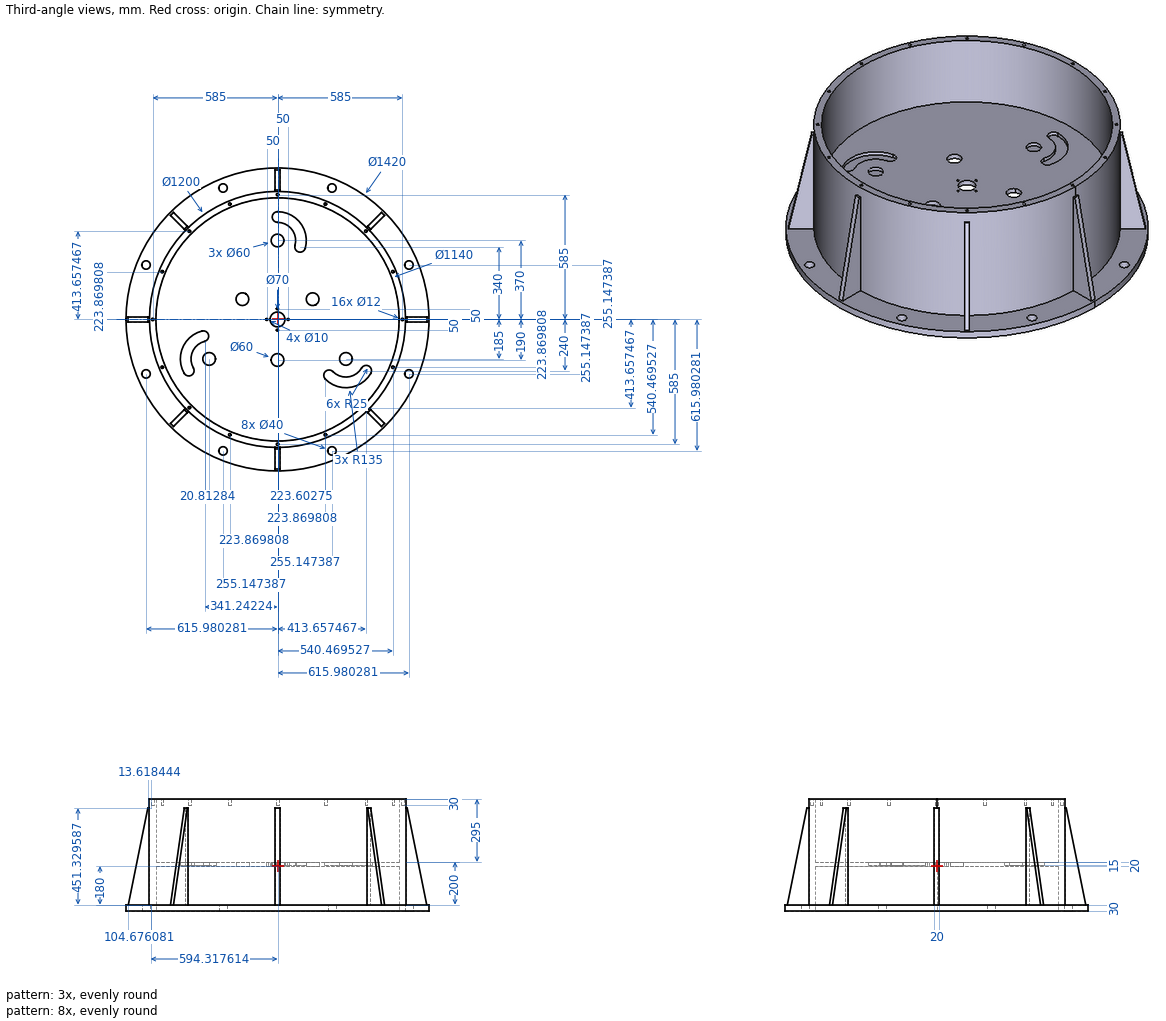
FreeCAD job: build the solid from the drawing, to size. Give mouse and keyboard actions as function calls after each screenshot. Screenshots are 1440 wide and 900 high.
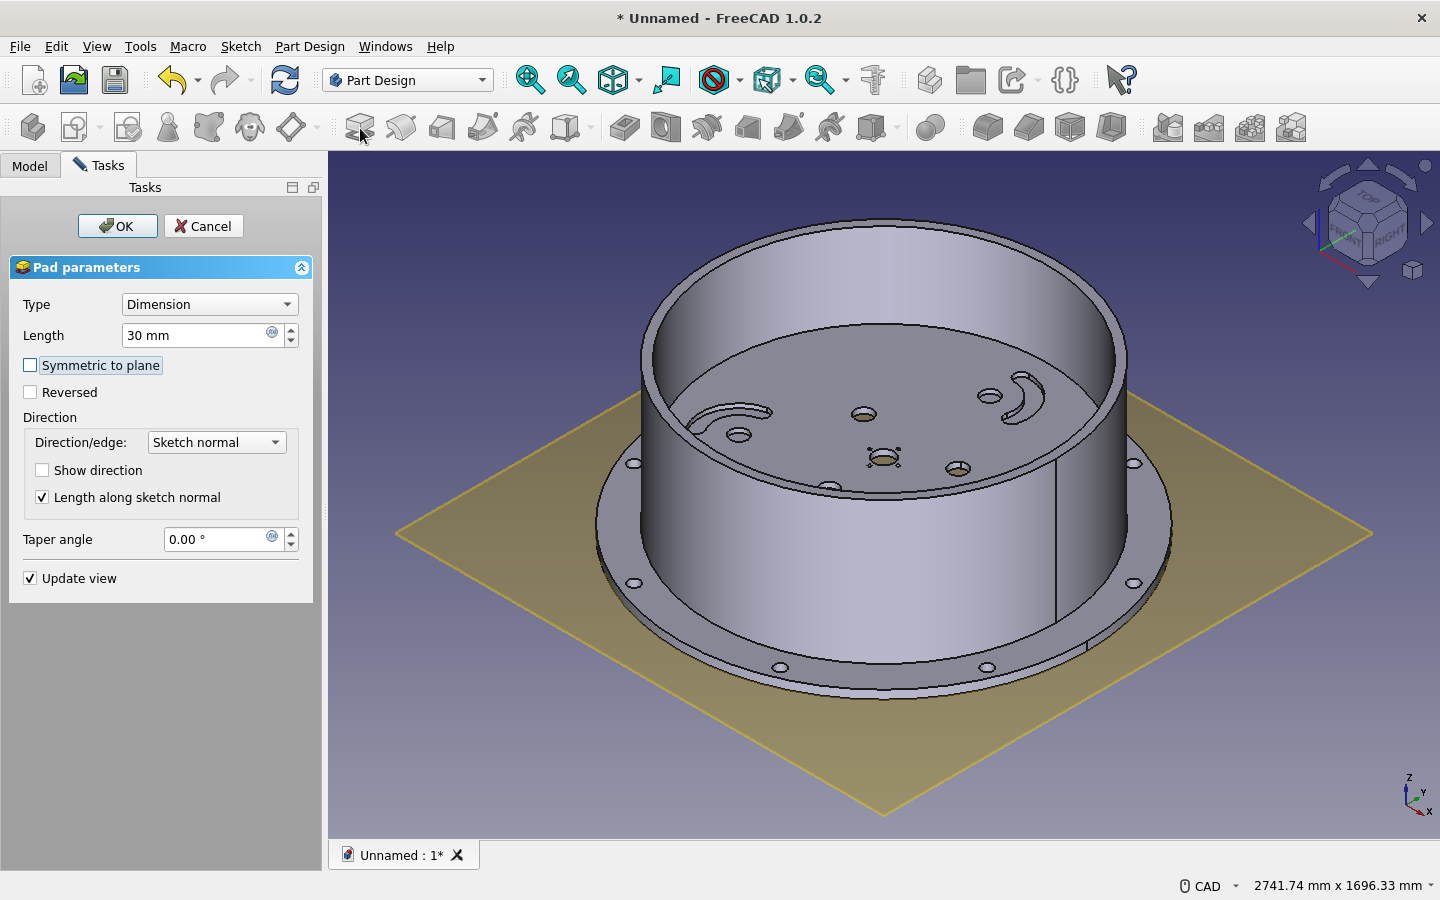
click(118, 226)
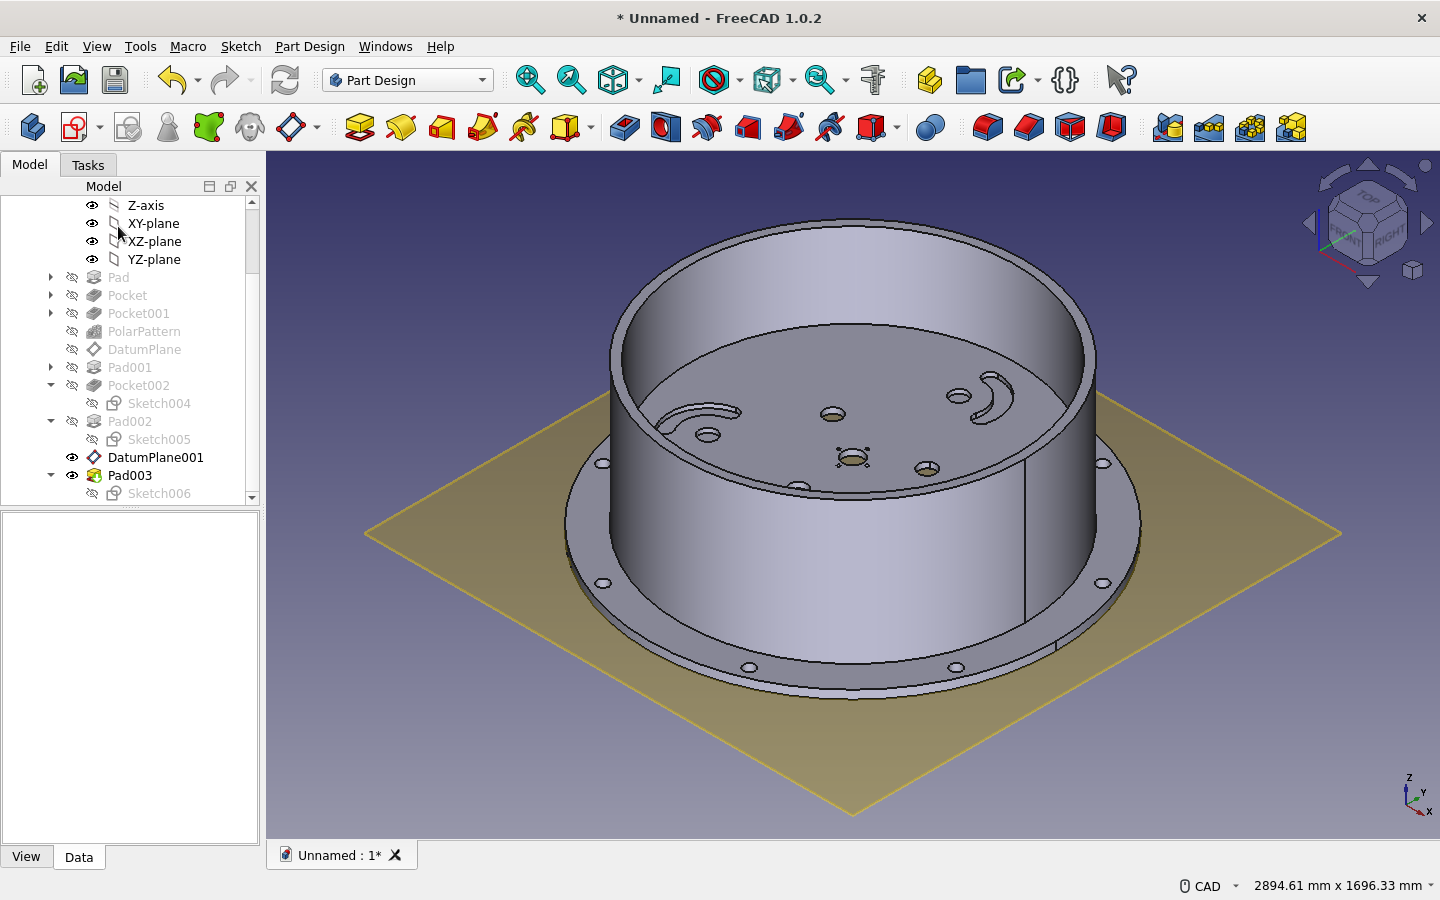
click(117, 457)
key(space)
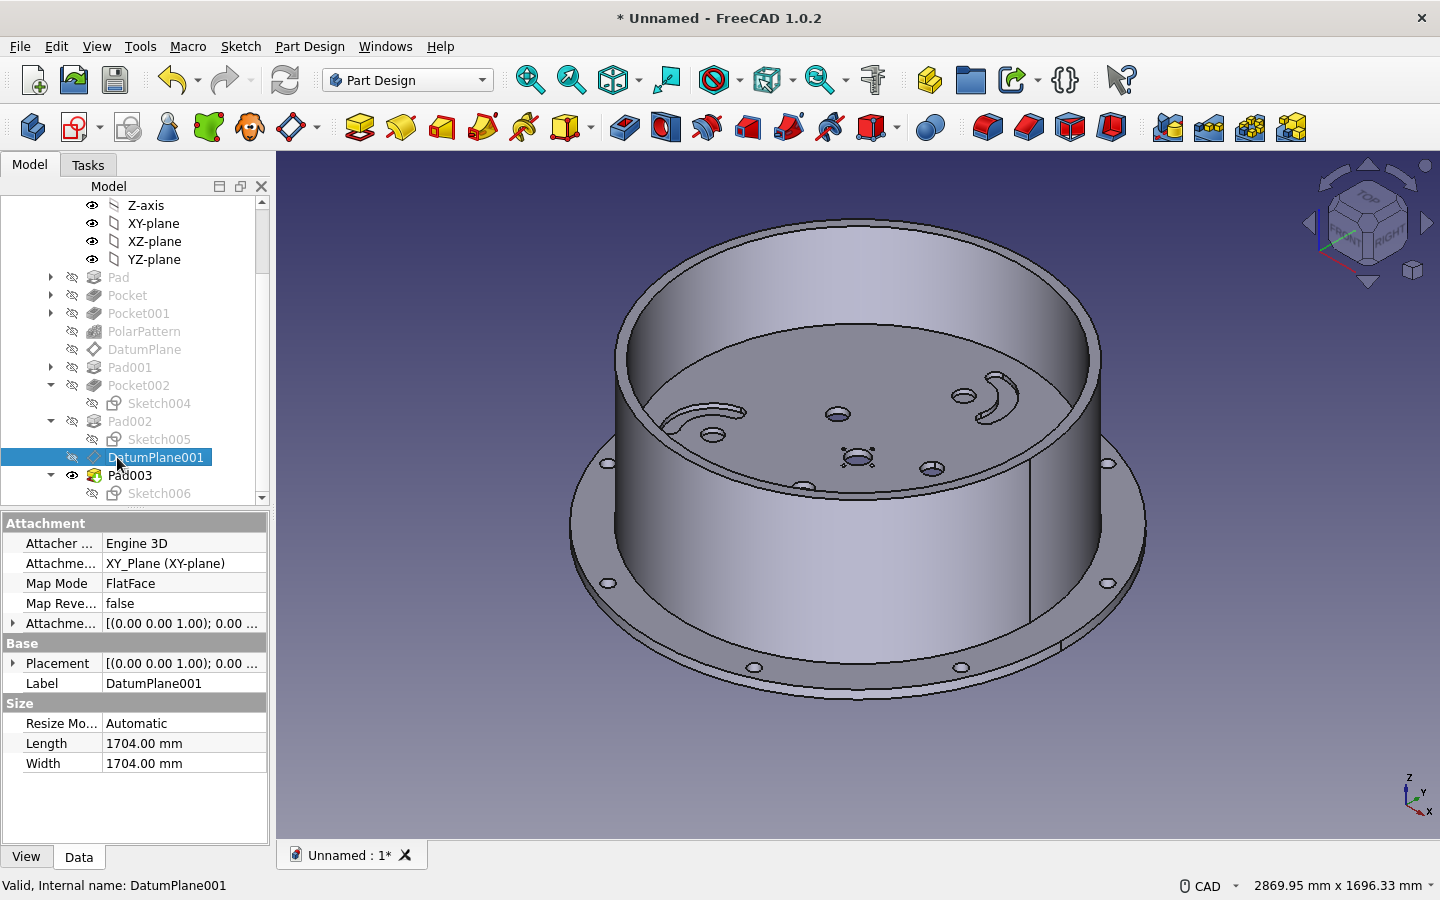
key(v)
key(f)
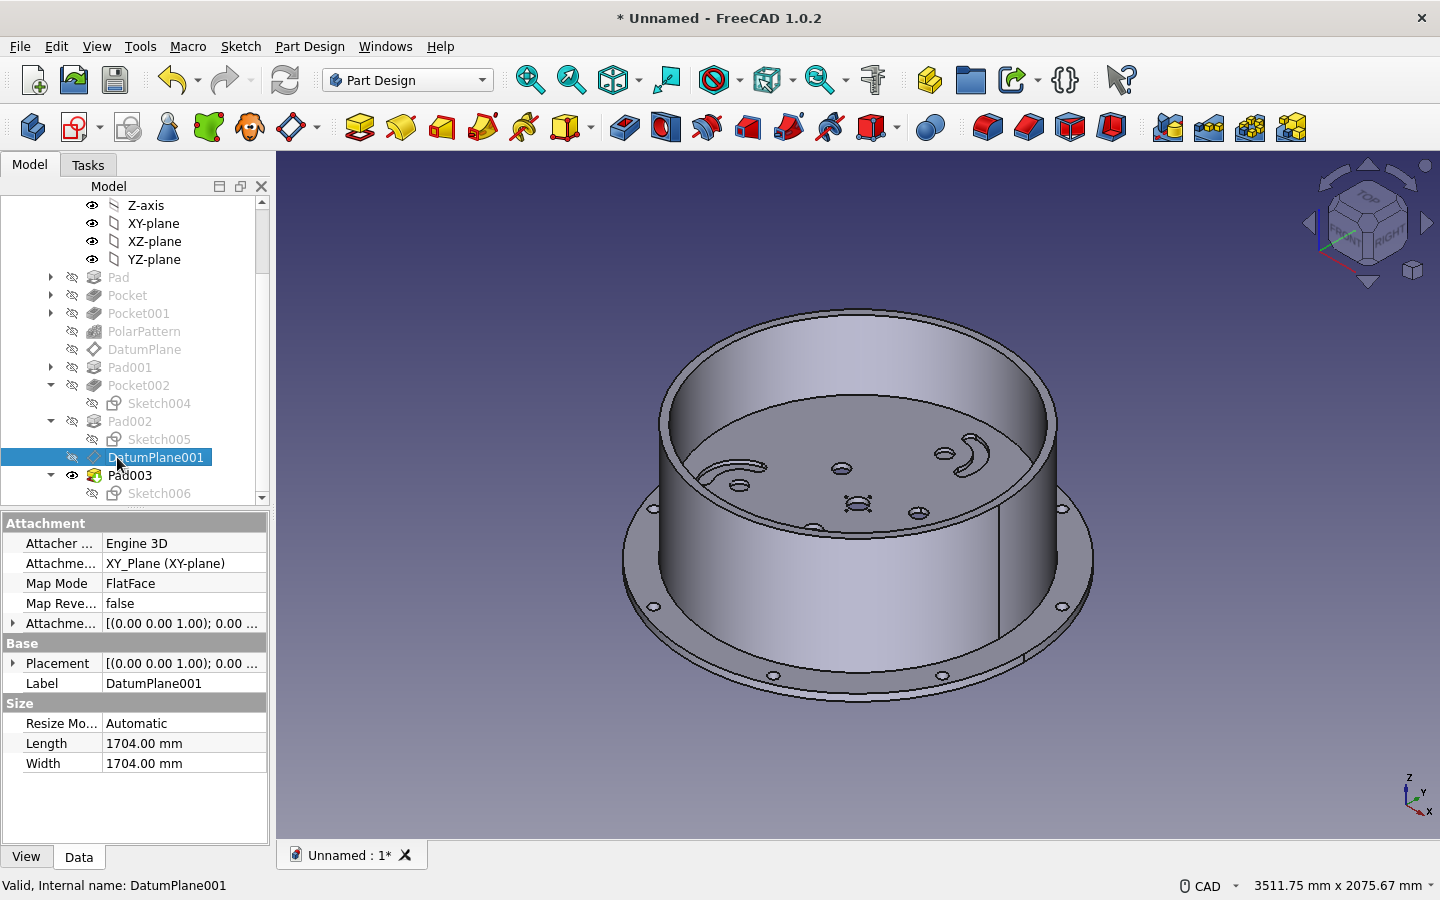
scroll(1027, 366, up, 7)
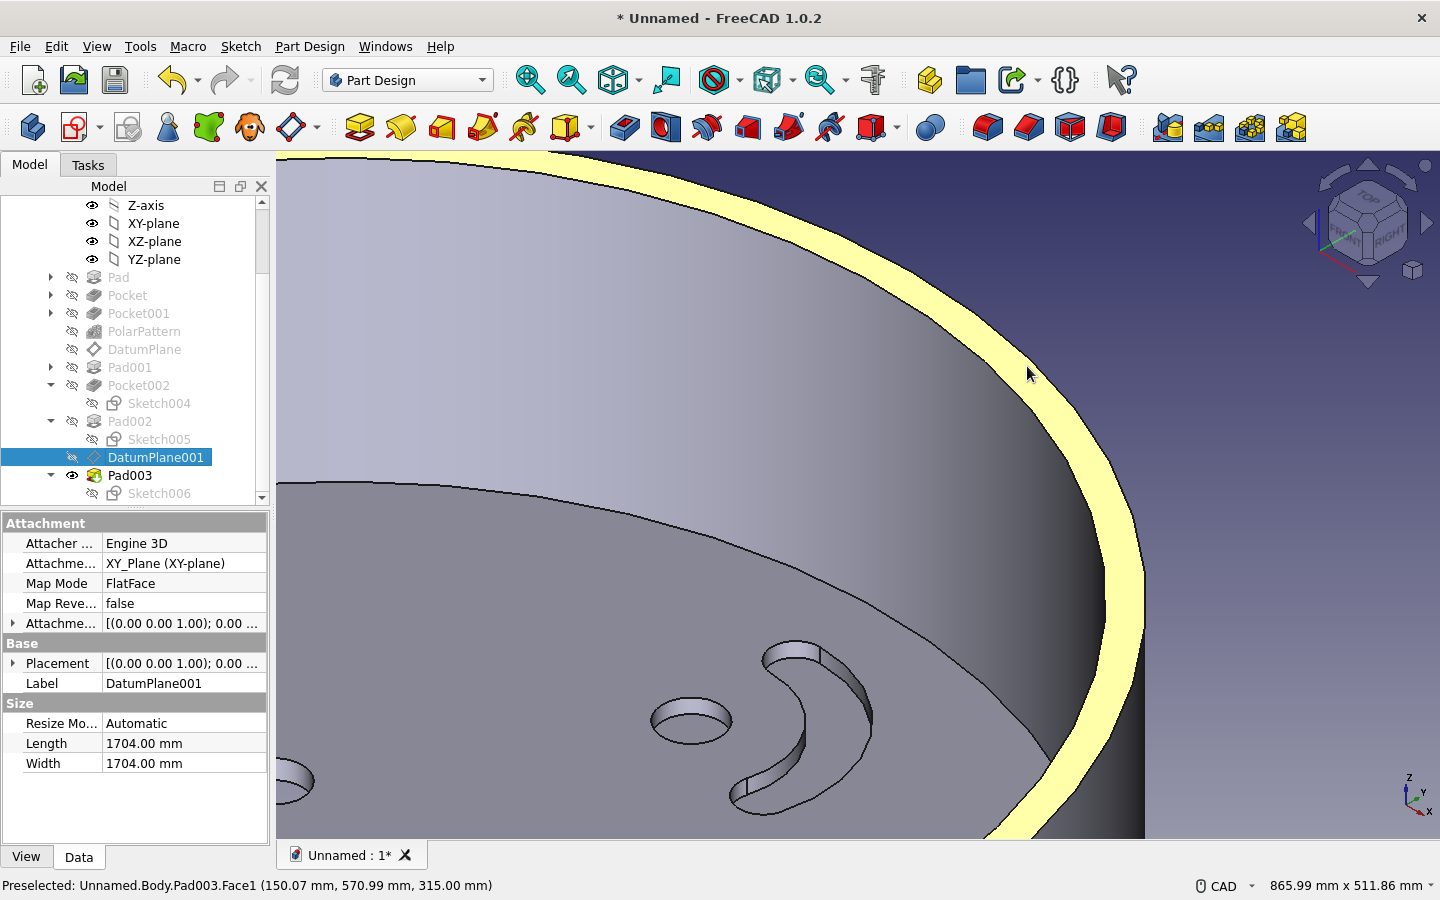
click(1025, 368)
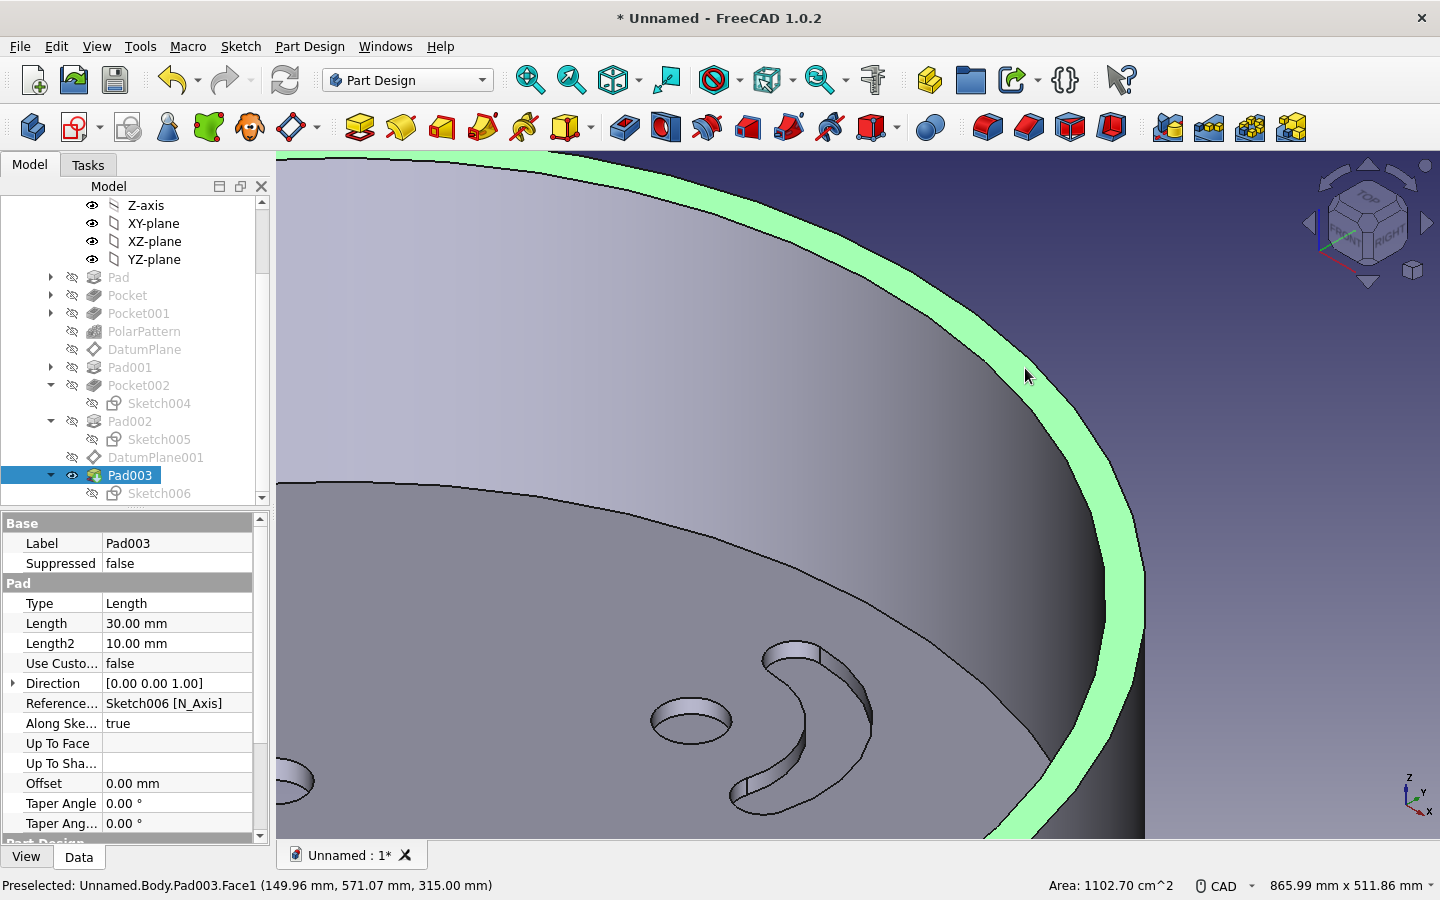
click(74, 128)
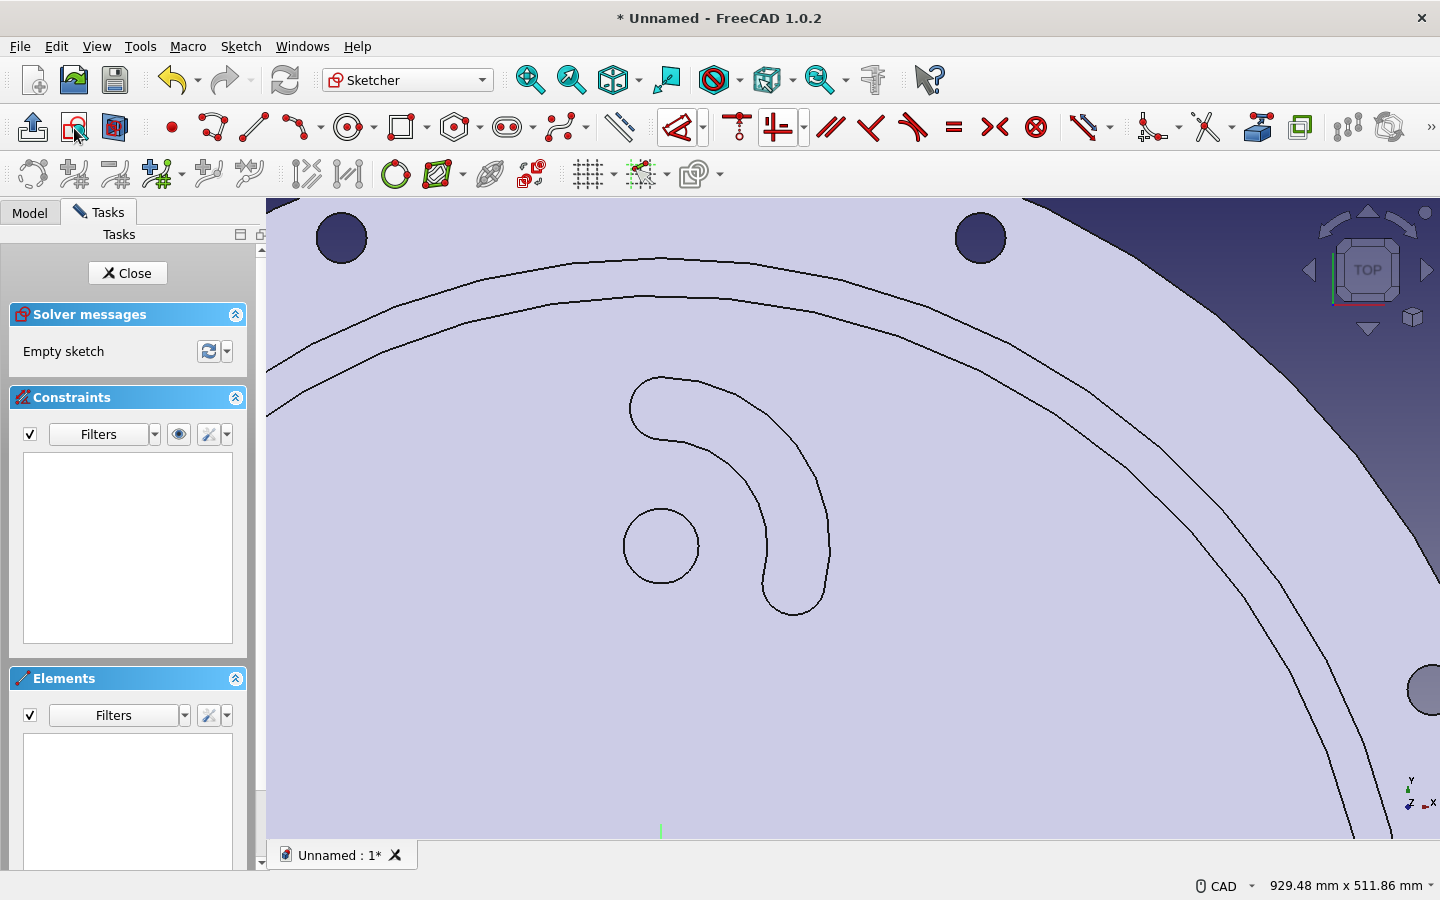
scroll(838, 307, down, 6)